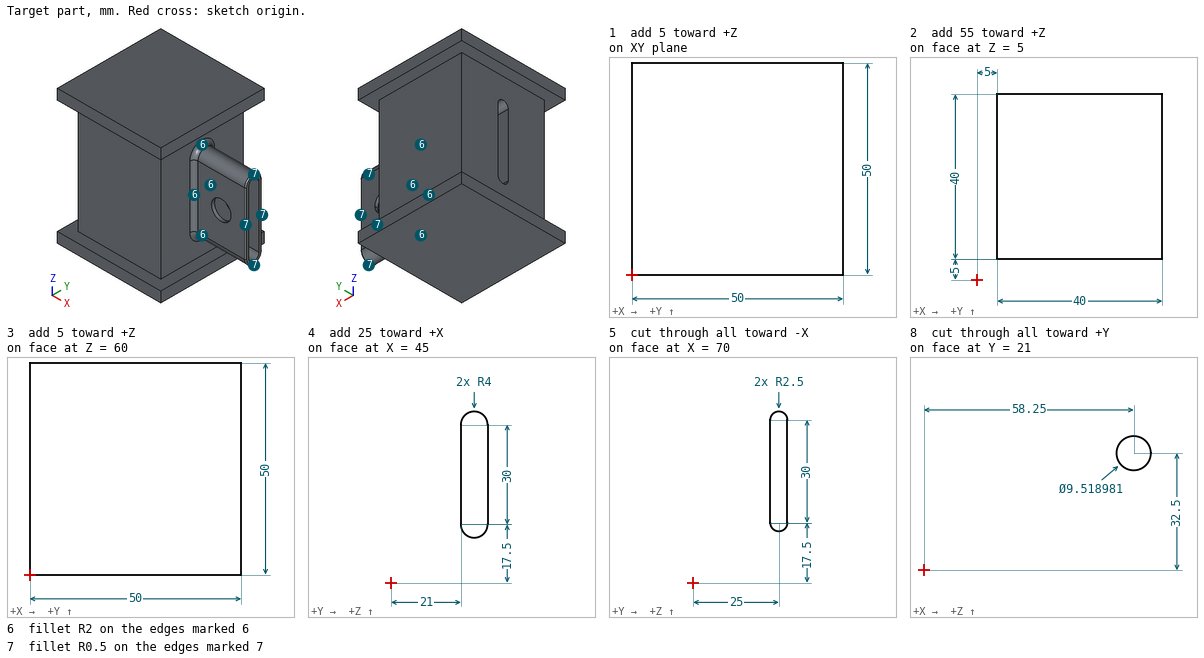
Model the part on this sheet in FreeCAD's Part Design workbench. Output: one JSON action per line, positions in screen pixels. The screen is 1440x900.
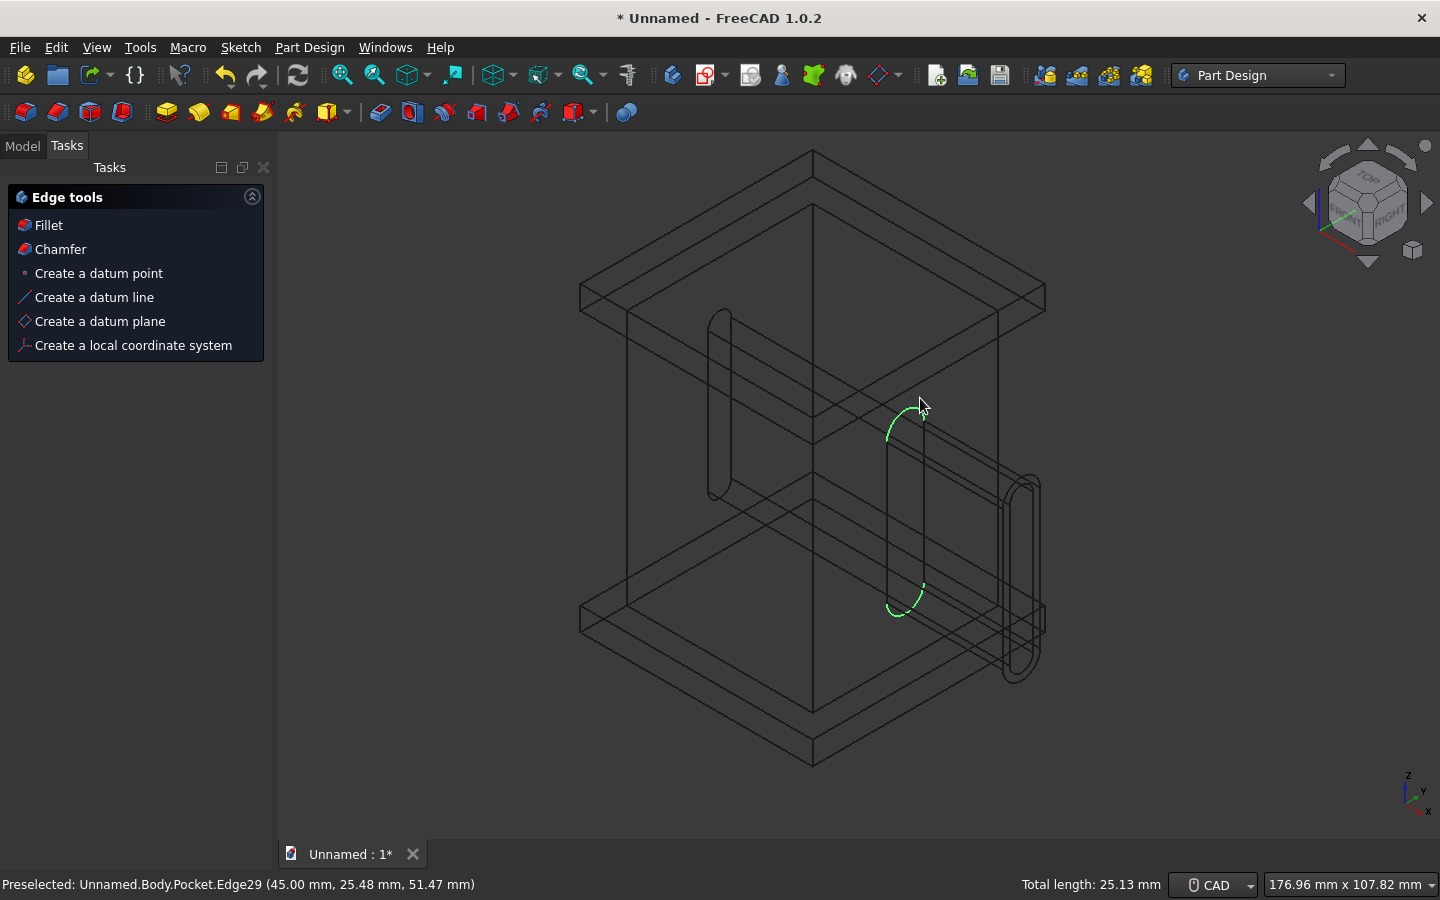
{"action": "left_click", "coordinate": [924, 500], "text": "ctrl"}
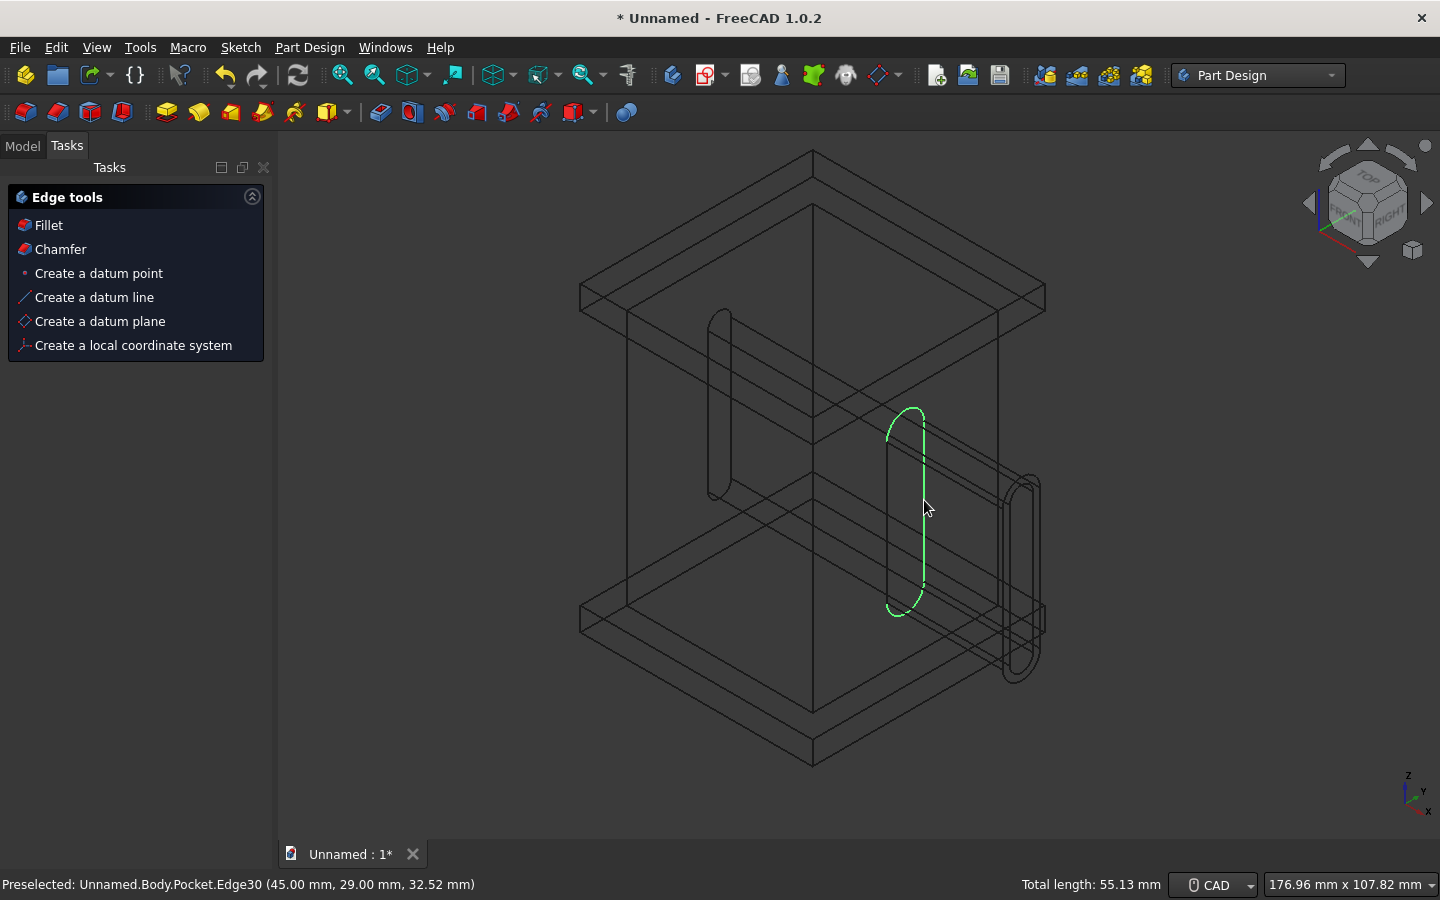
{"action": "left_click", "coordinate": [887, 522], "text": "ctrl"}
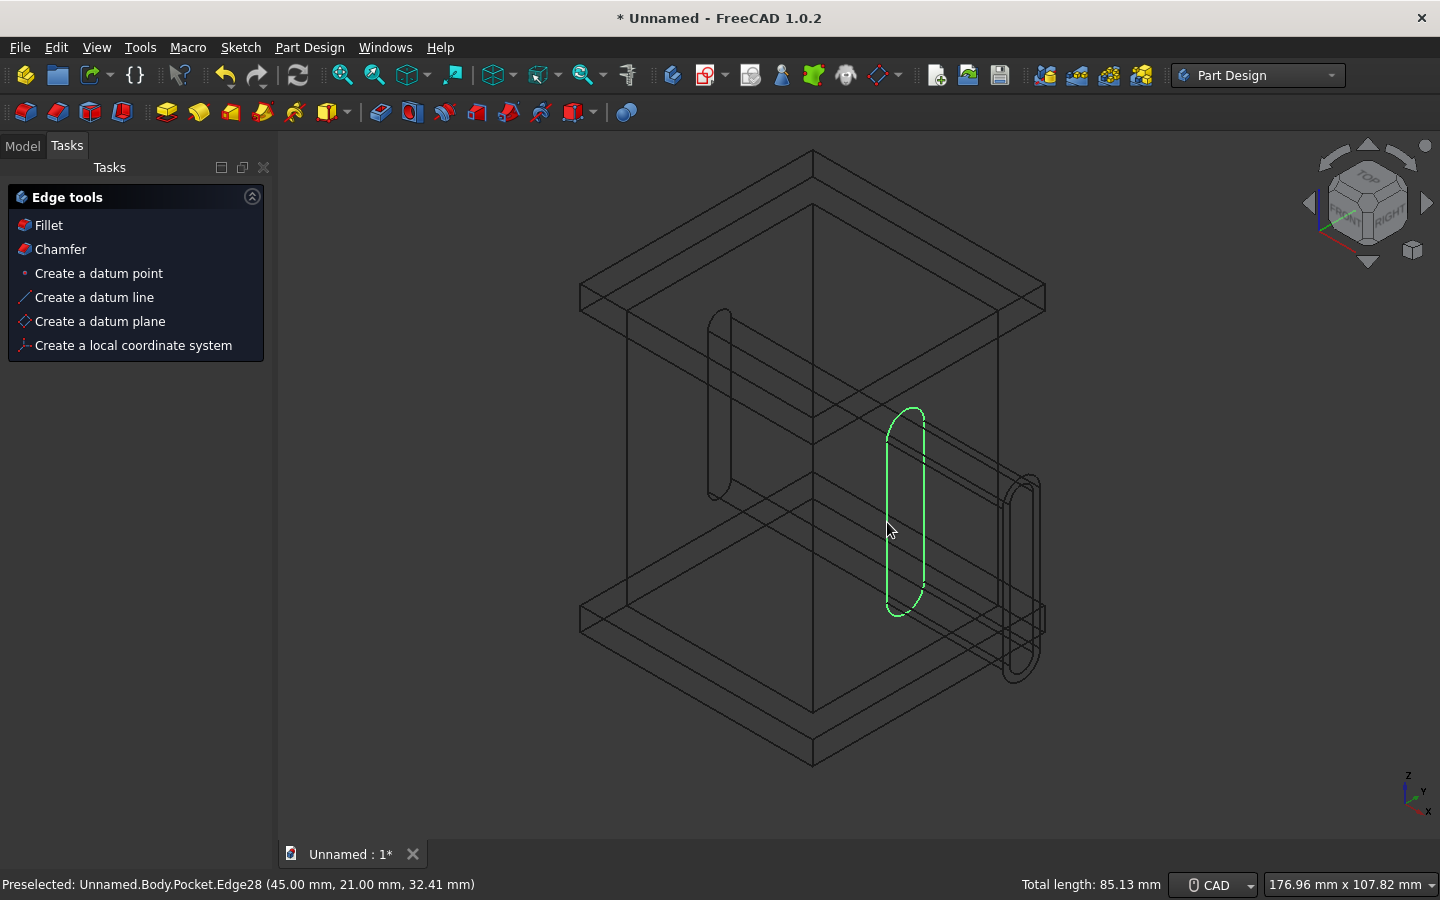
{"action": "key", "text": "v 1"}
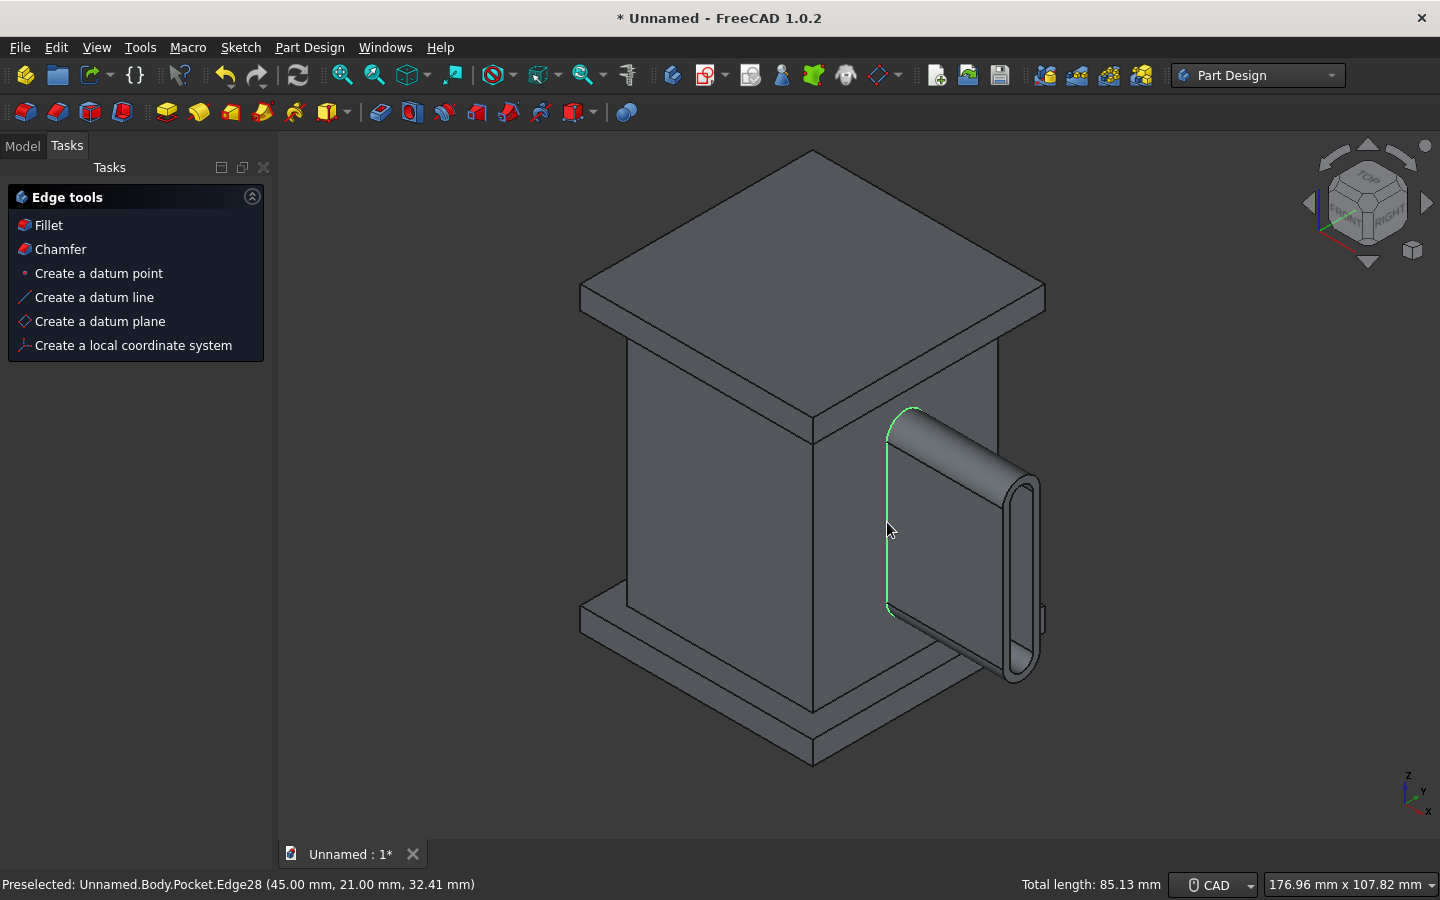
{"action": "left_click", "coordinate": [26, 112]}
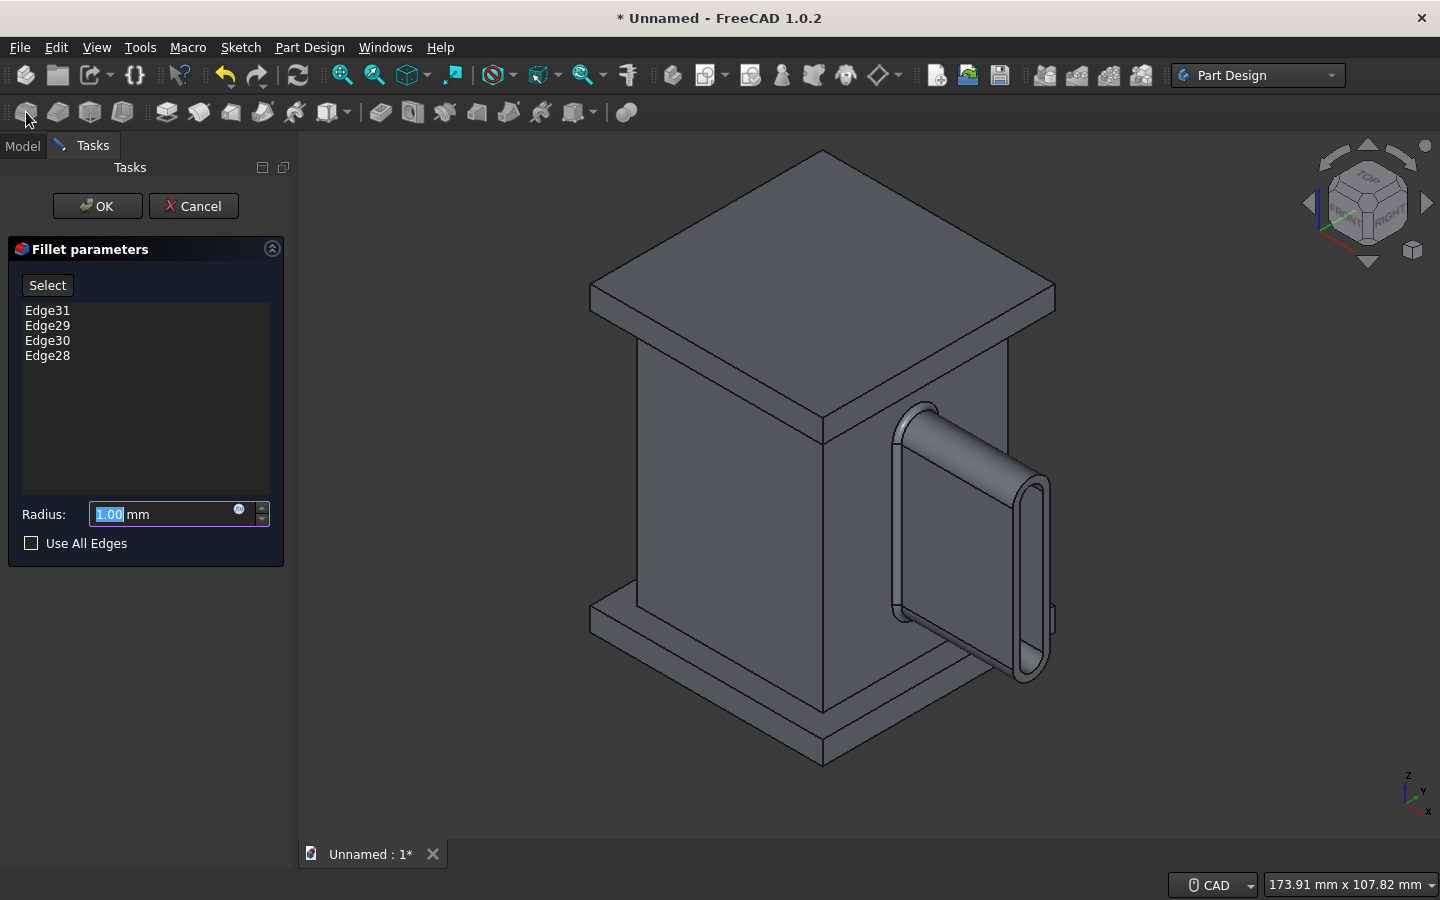
{"action": "type", "text": "2"}
{"action": "key", "text": "Tab"}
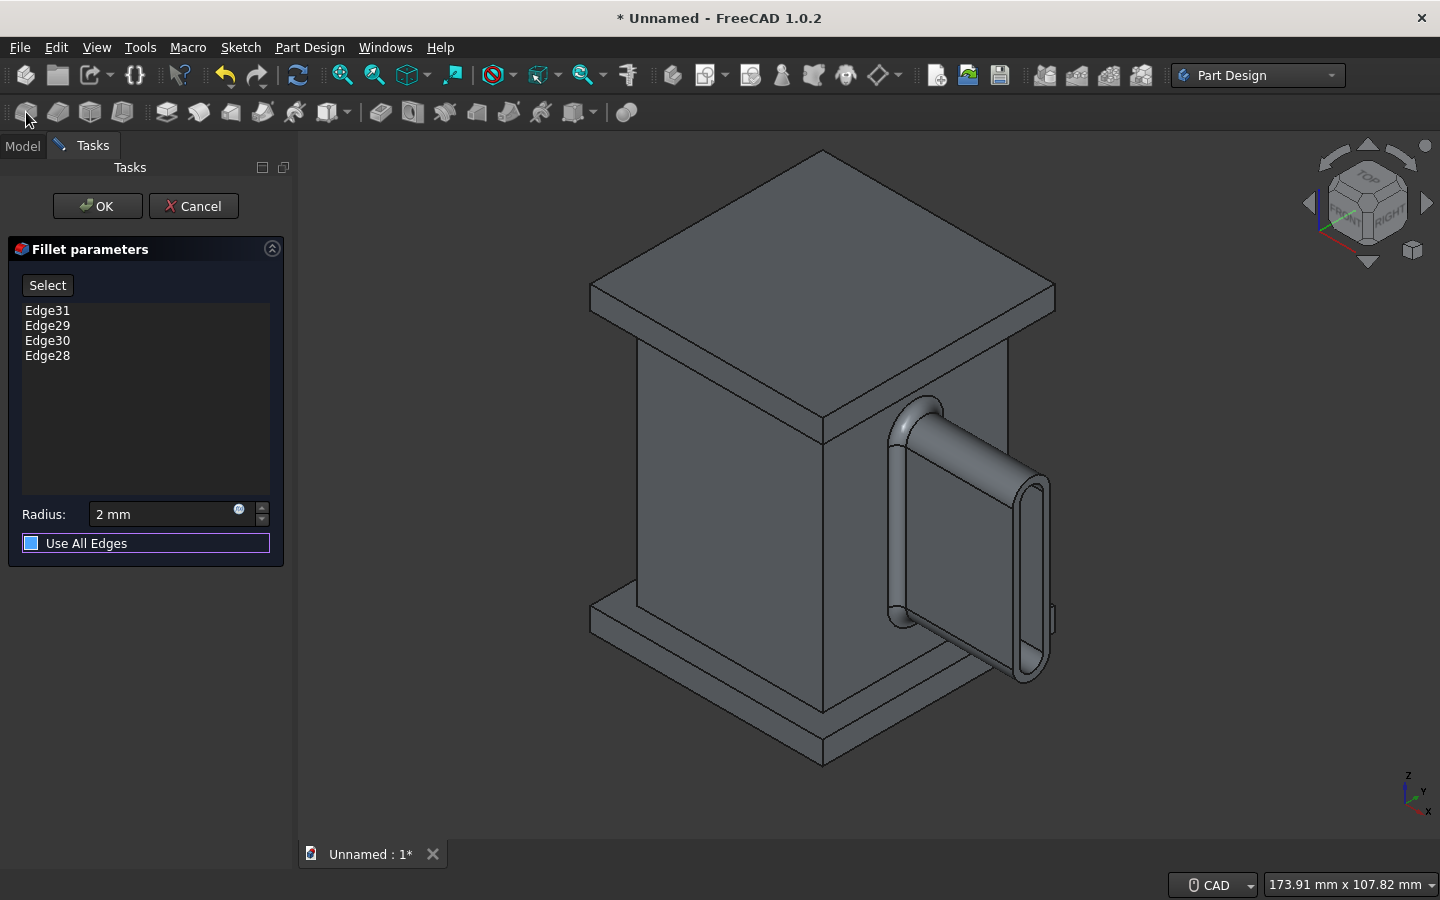
{"action": "left_click", "coordinate": [98, 206]}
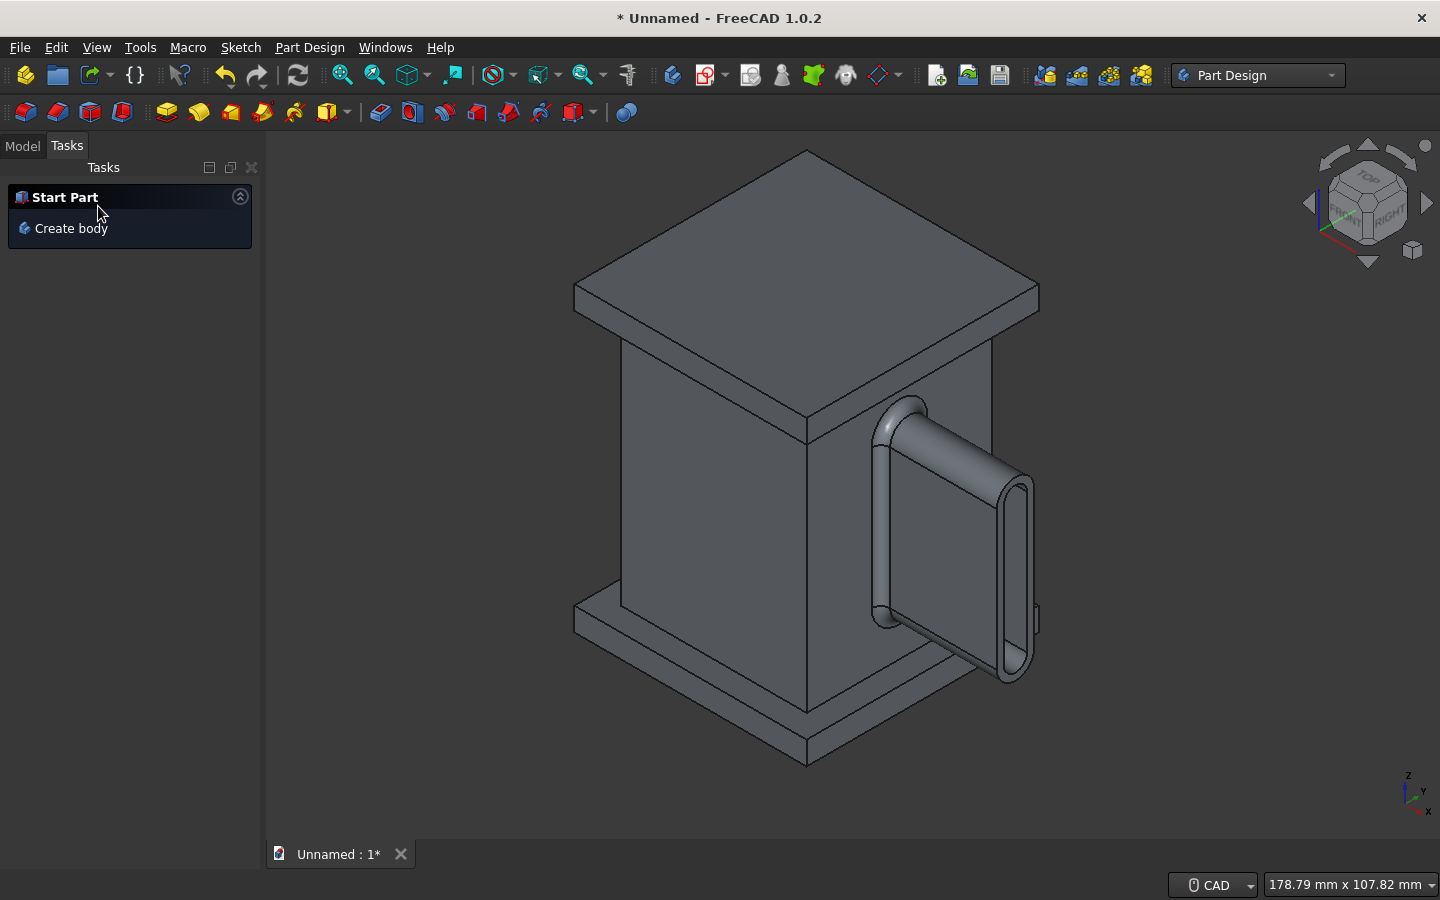
{"action": "left_click", "coordinate": [997, 589]}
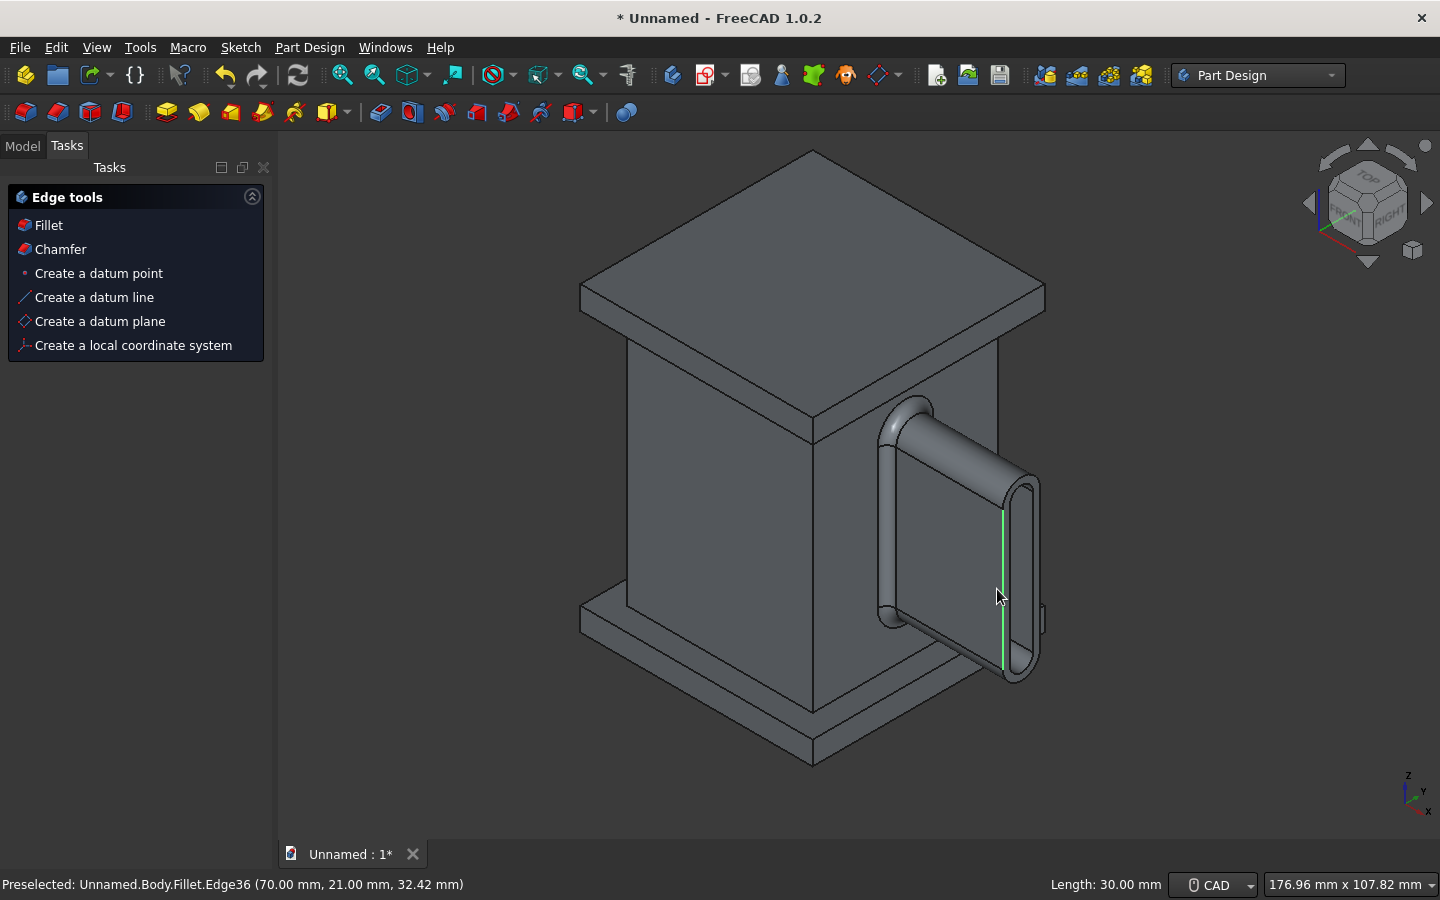
{"action": "left_click", "coordinate": [1022, 680], "text": "ctrl"}